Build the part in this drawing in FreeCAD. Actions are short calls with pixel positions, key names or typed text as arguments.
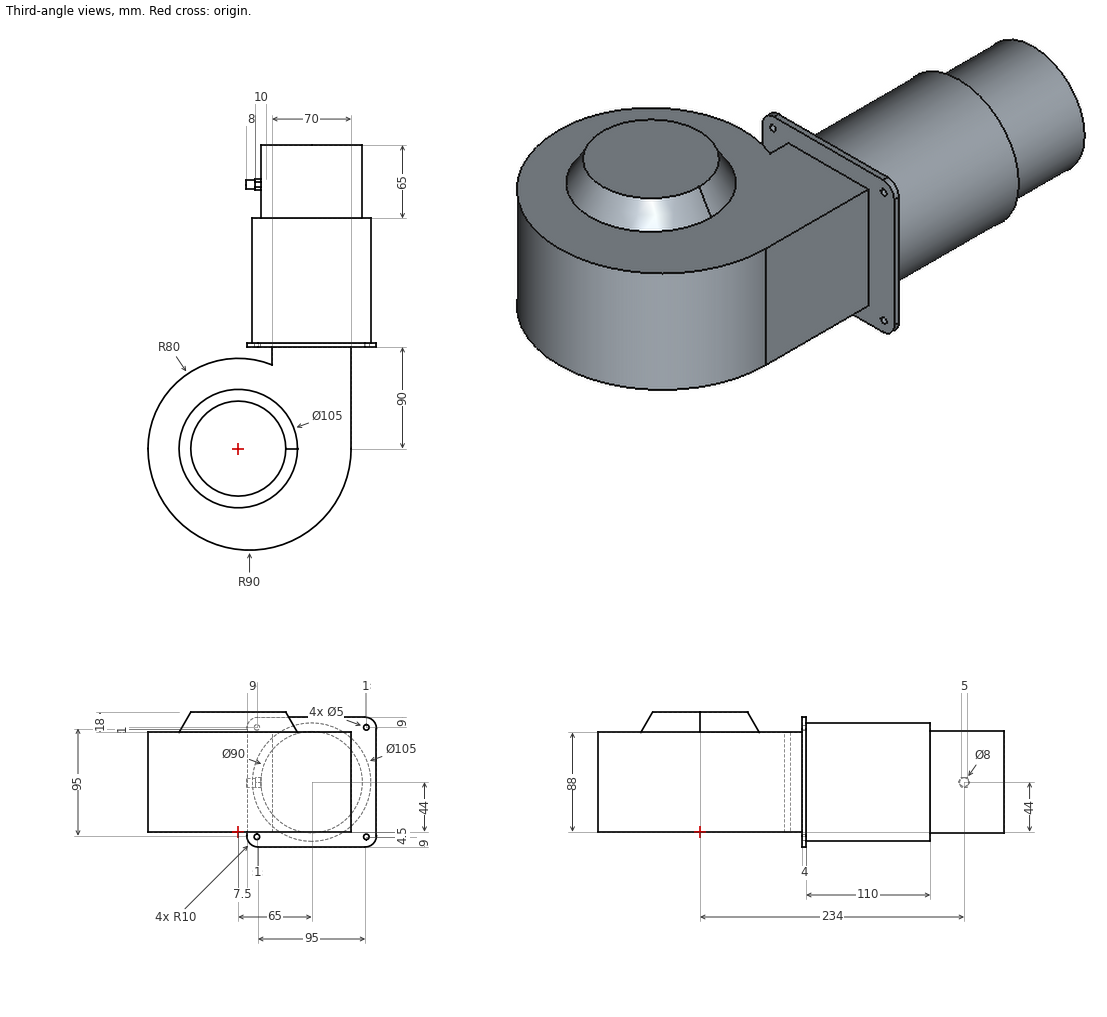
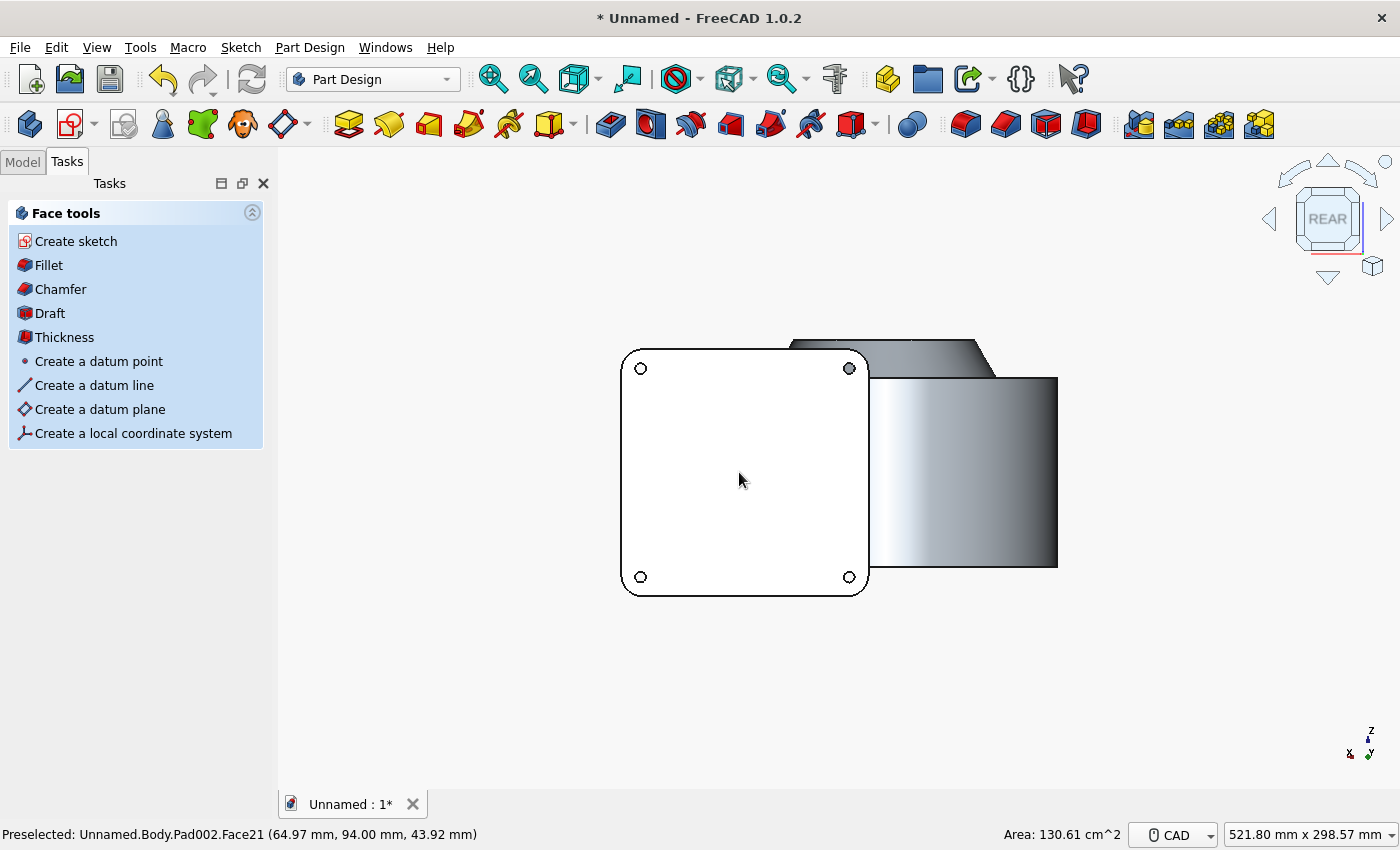
click(70, 124)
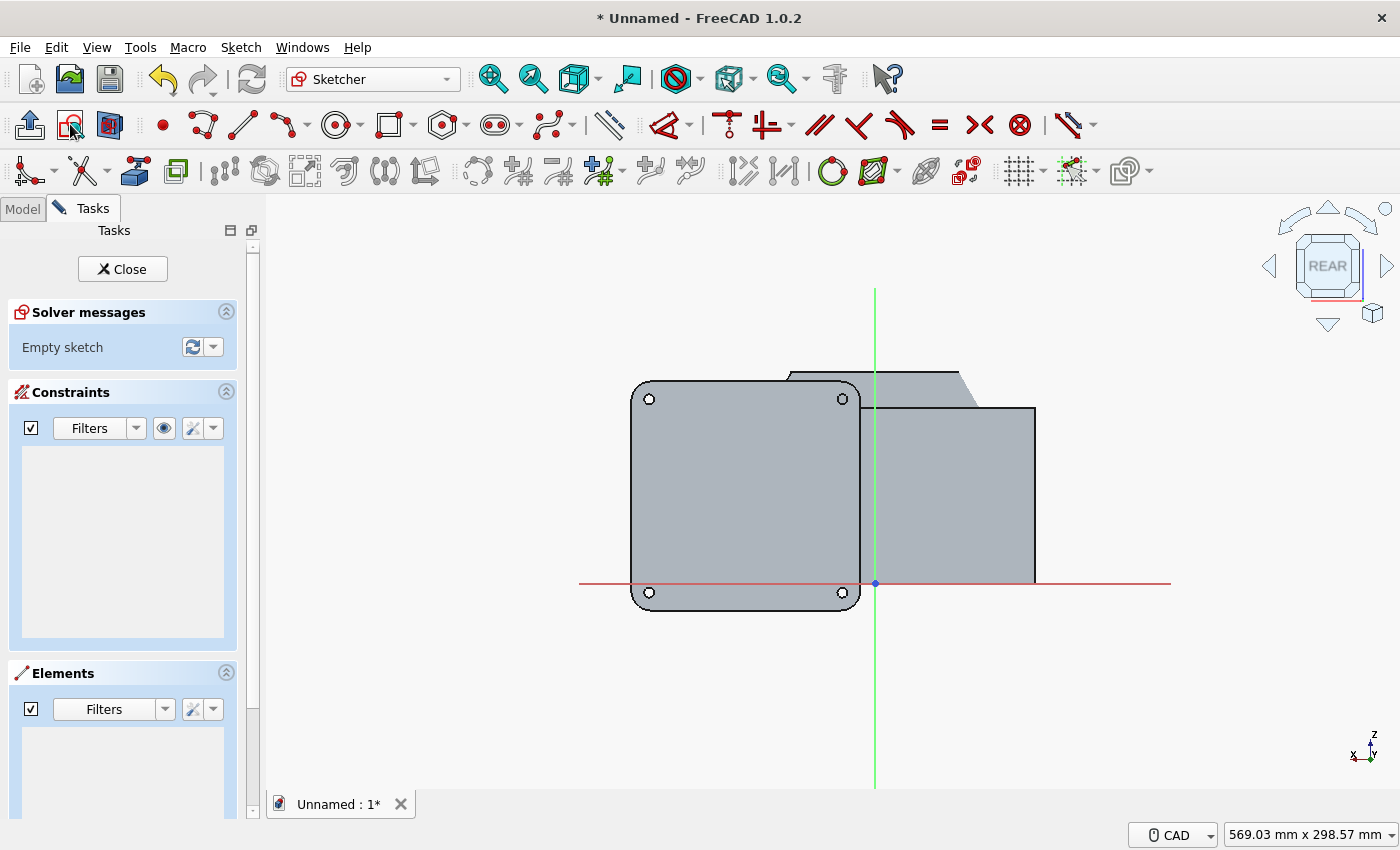
scroll(751, 501, up, 3)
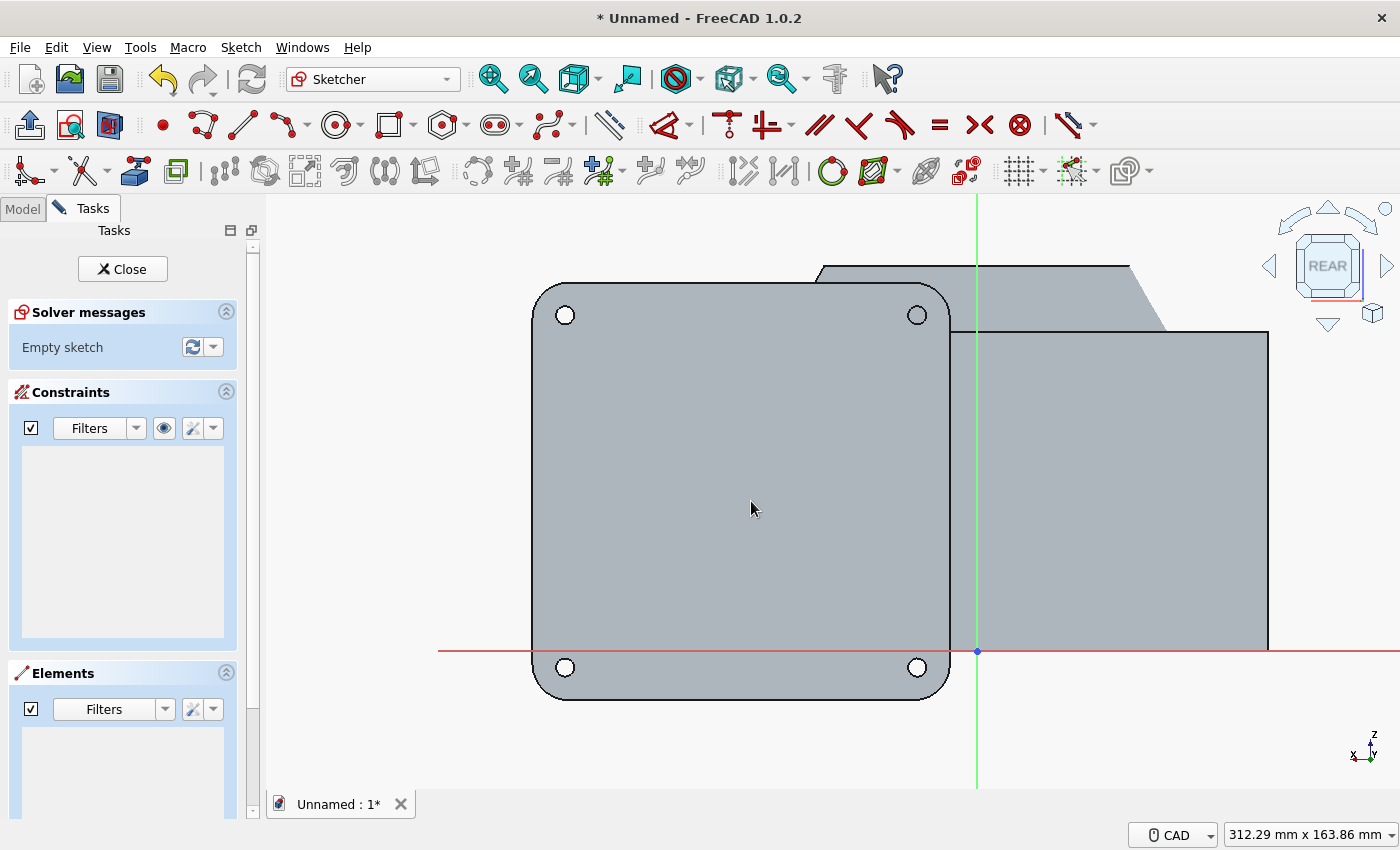
click(336, 126)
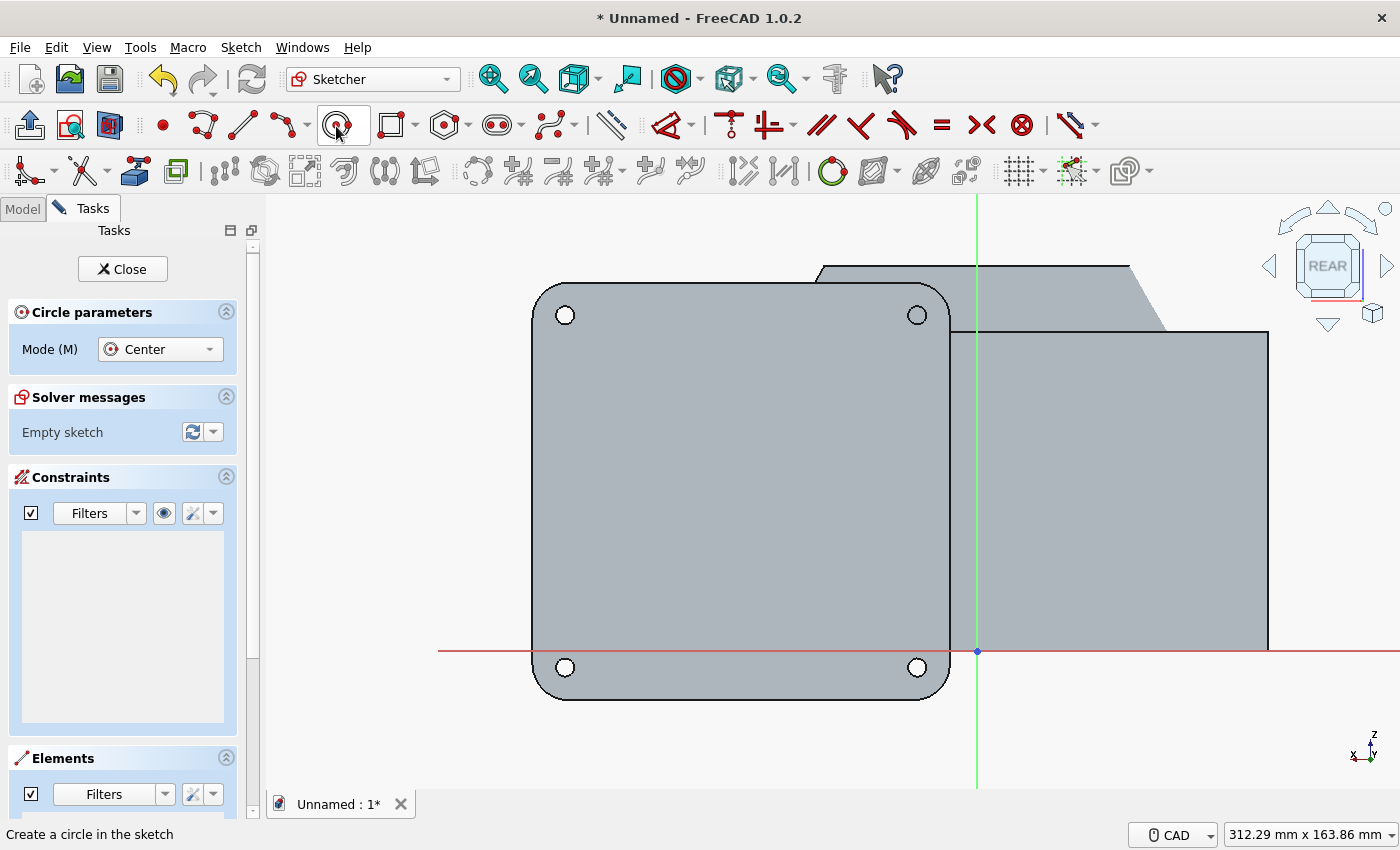
click(741, 491)
click(876, 357)
key(Escape)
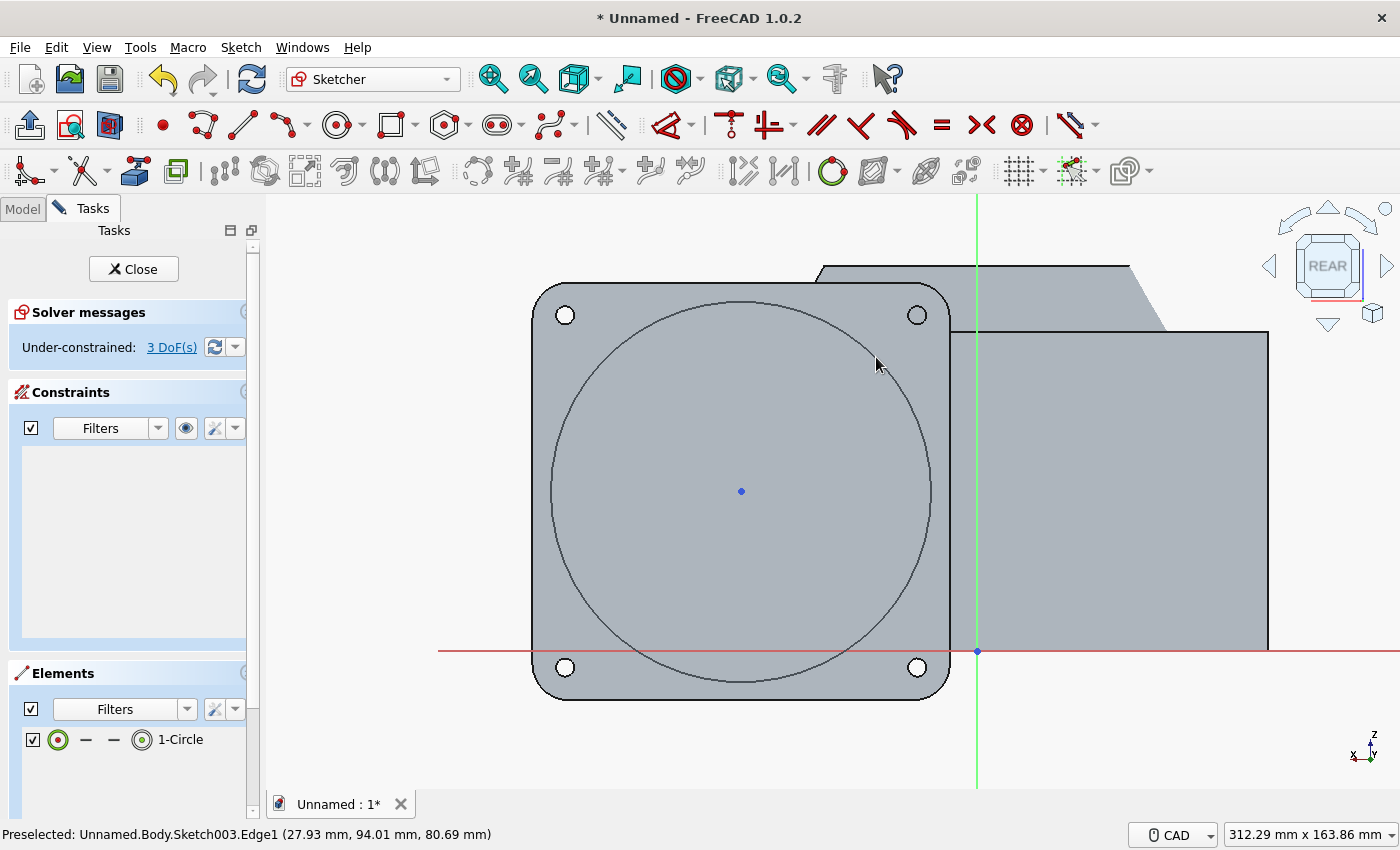
click(666, 126)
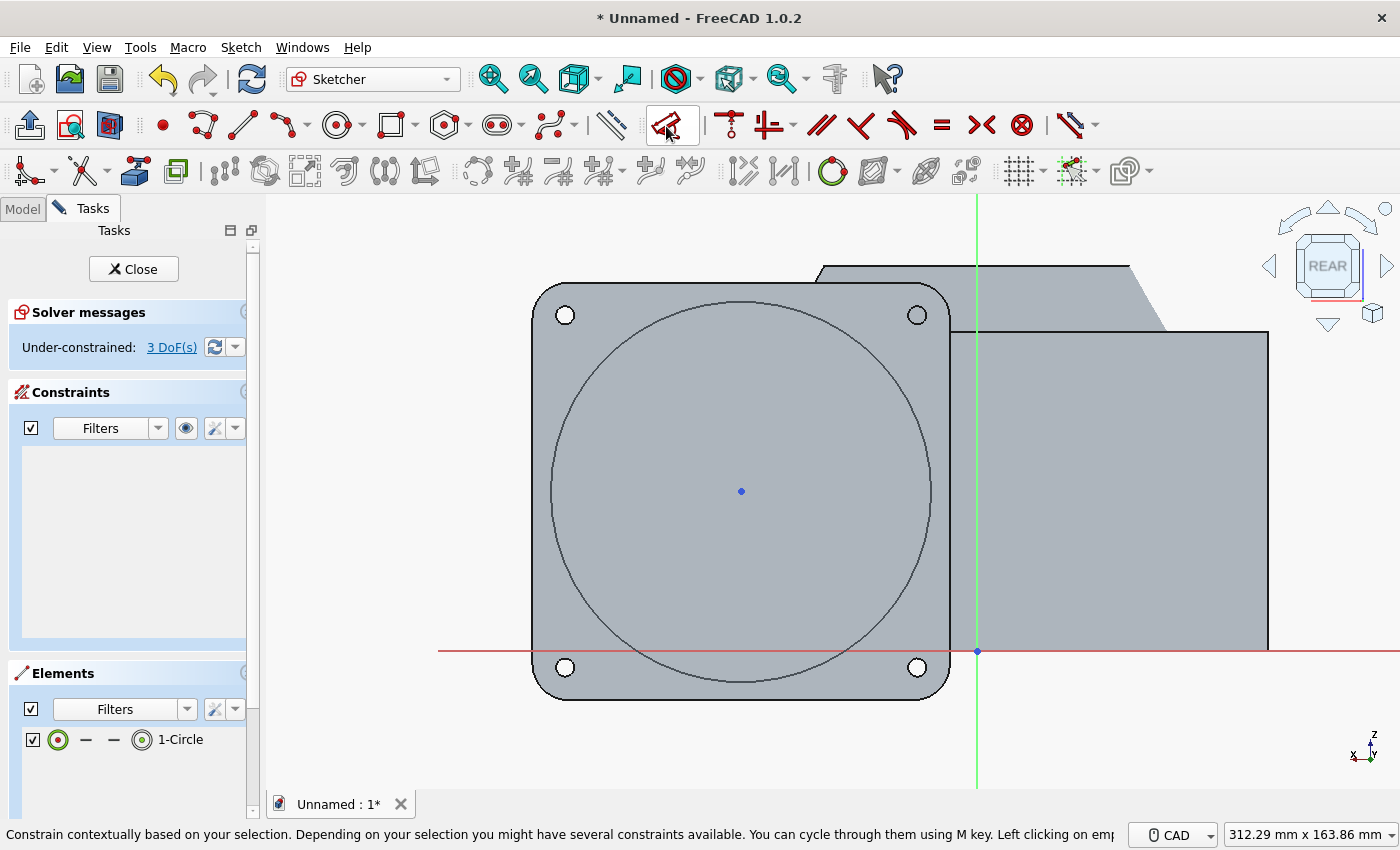
click(875, 357)
click(898, 334)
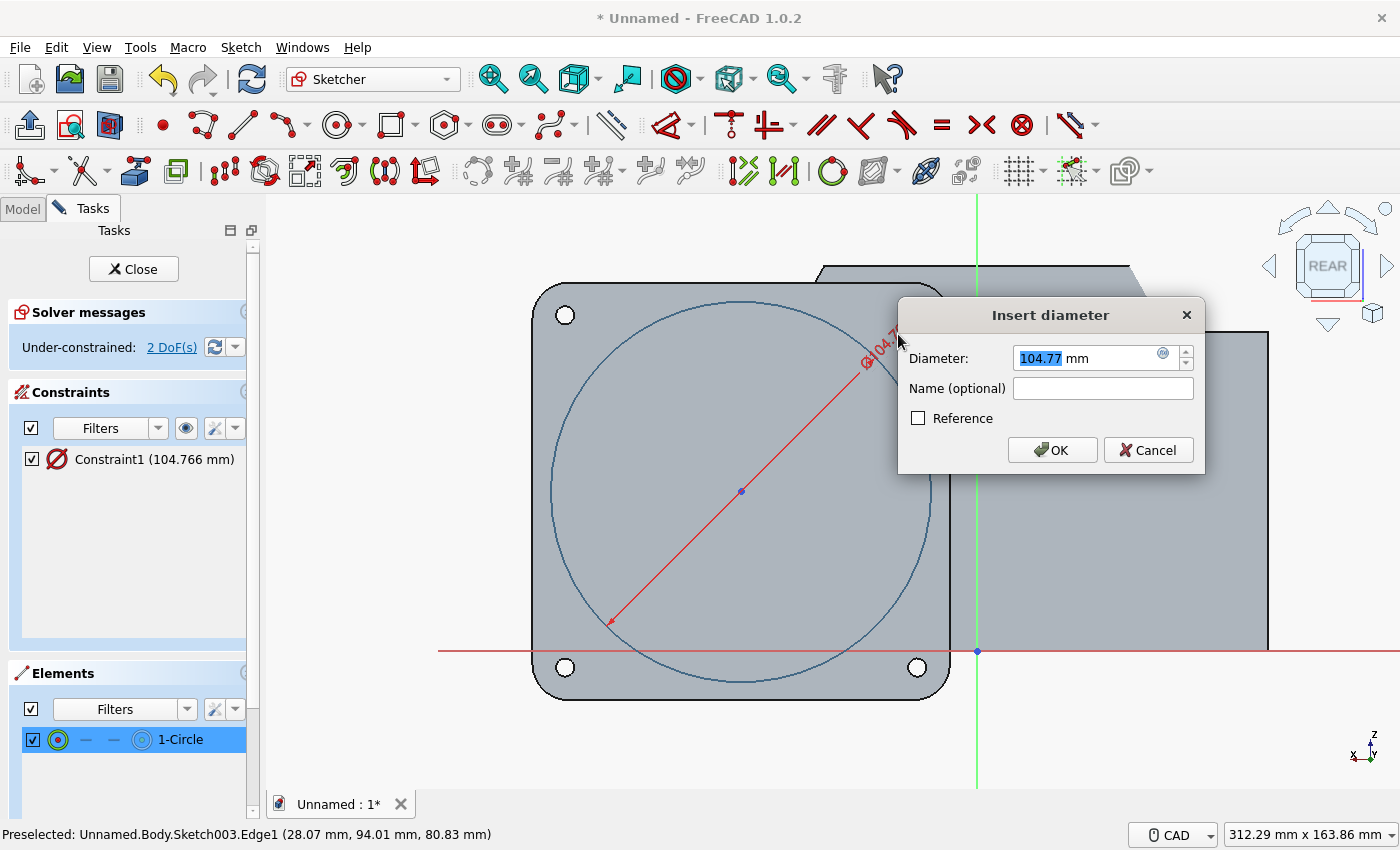
text(105)
key(Return)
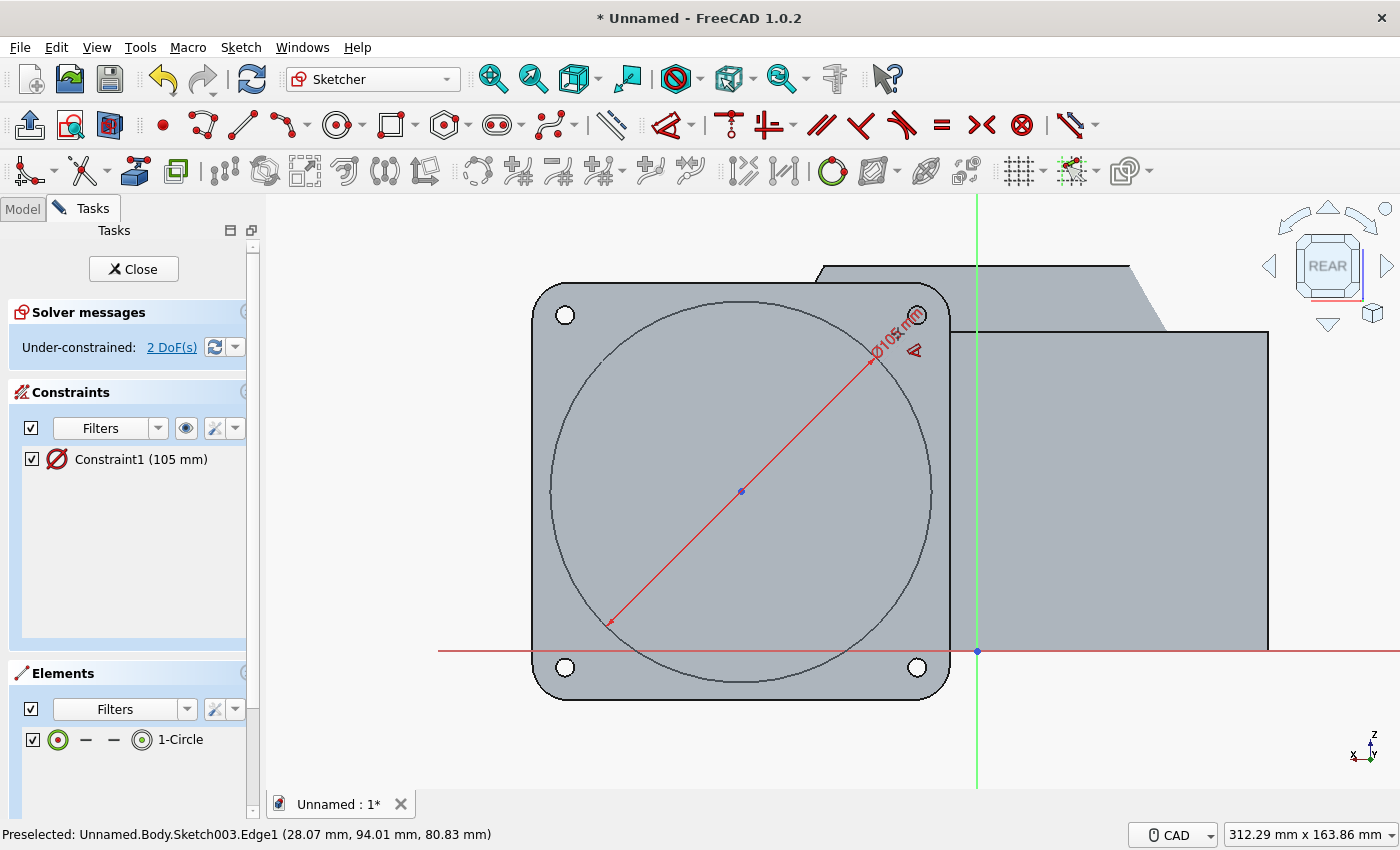
click(741, 492)
click(859, 685)